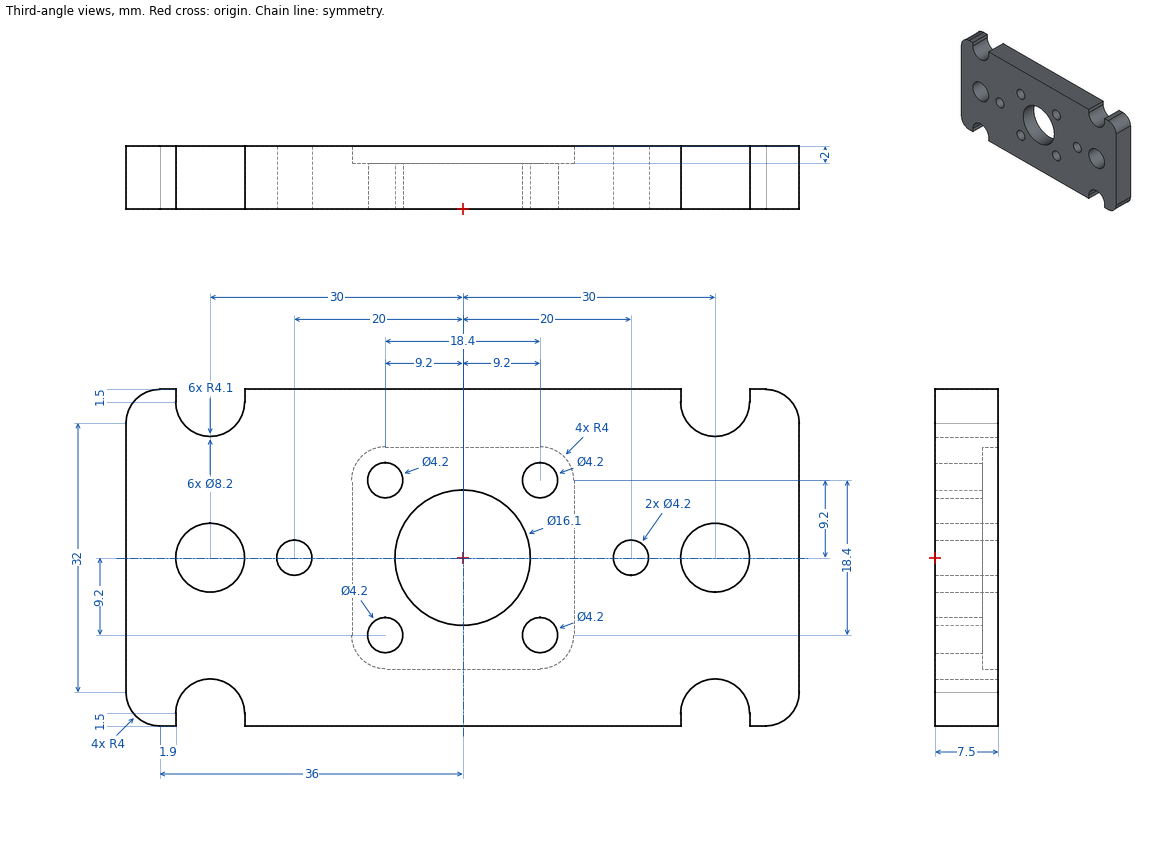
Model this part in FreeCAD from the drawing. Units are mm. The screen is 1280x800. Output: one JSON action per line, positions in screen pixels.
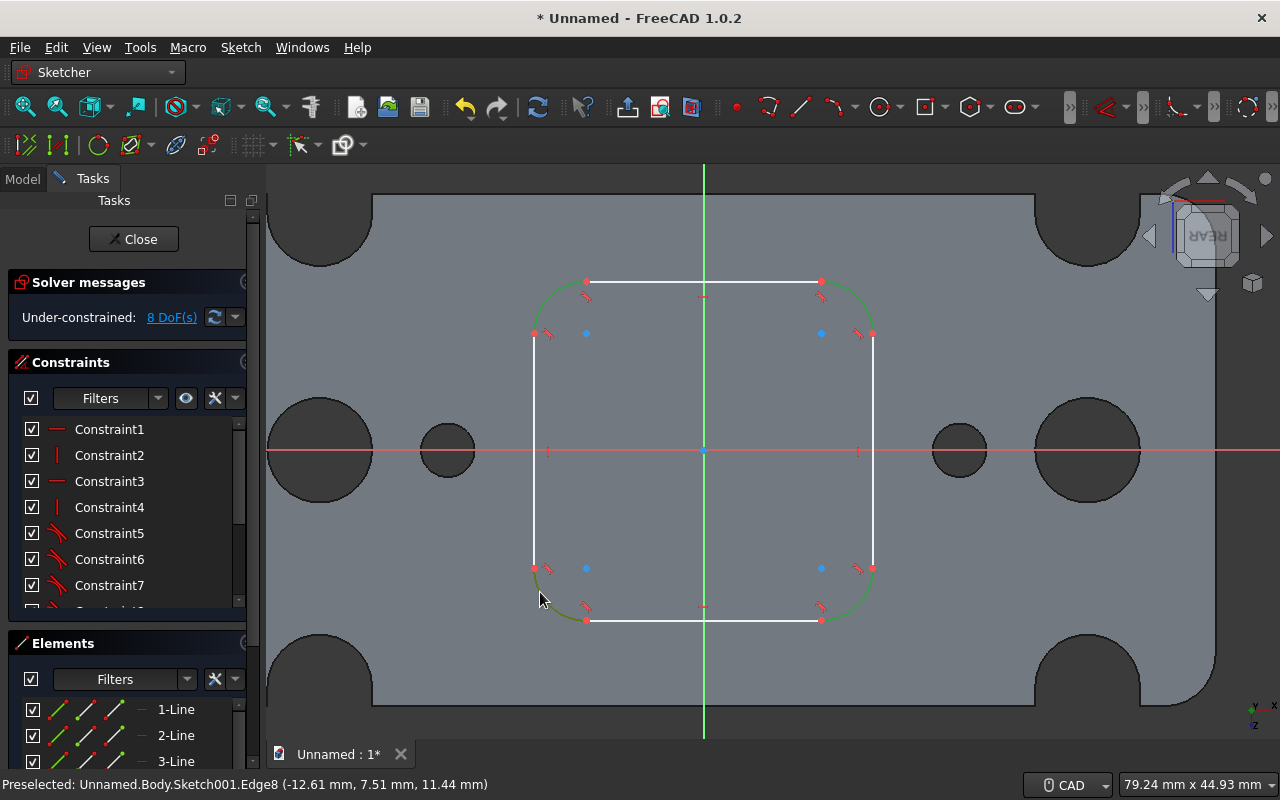
{"action": "key", "text": "e"}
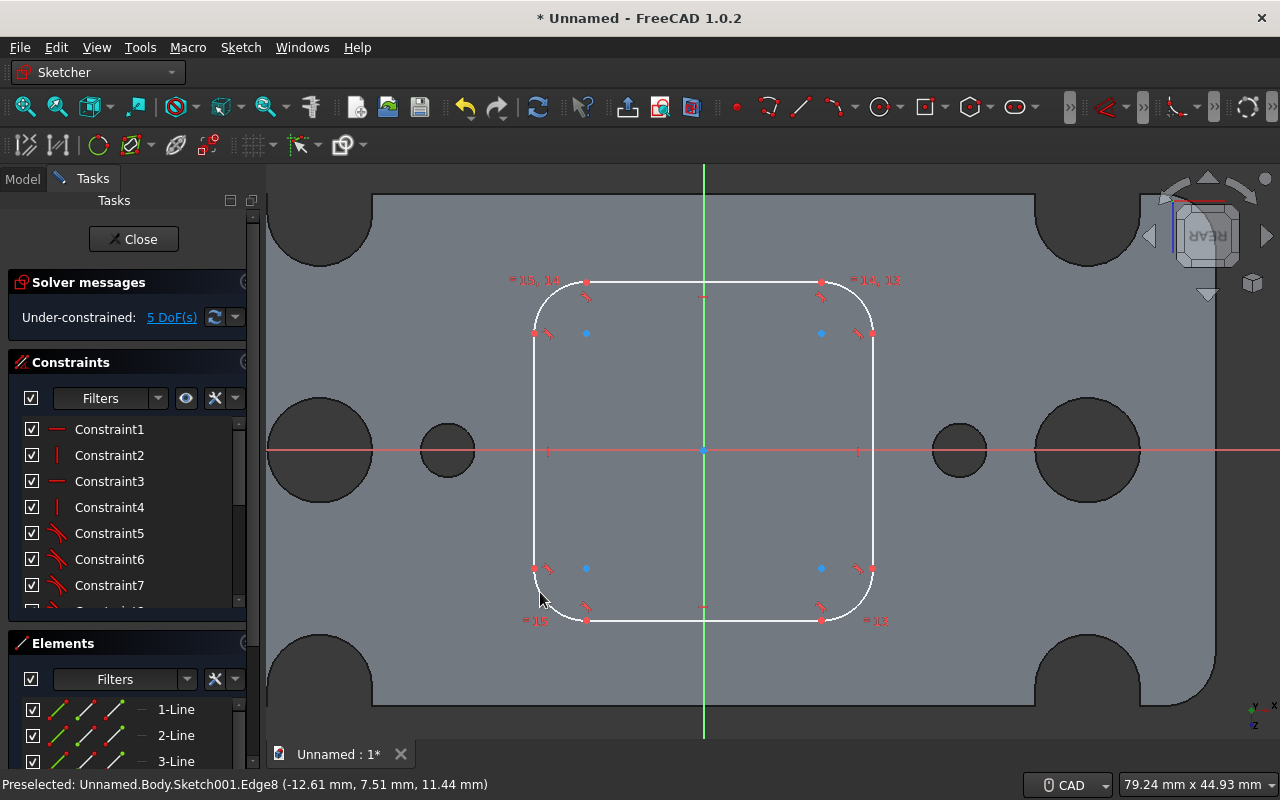
{"action": "left_click", "coordinate": [1106, 108]}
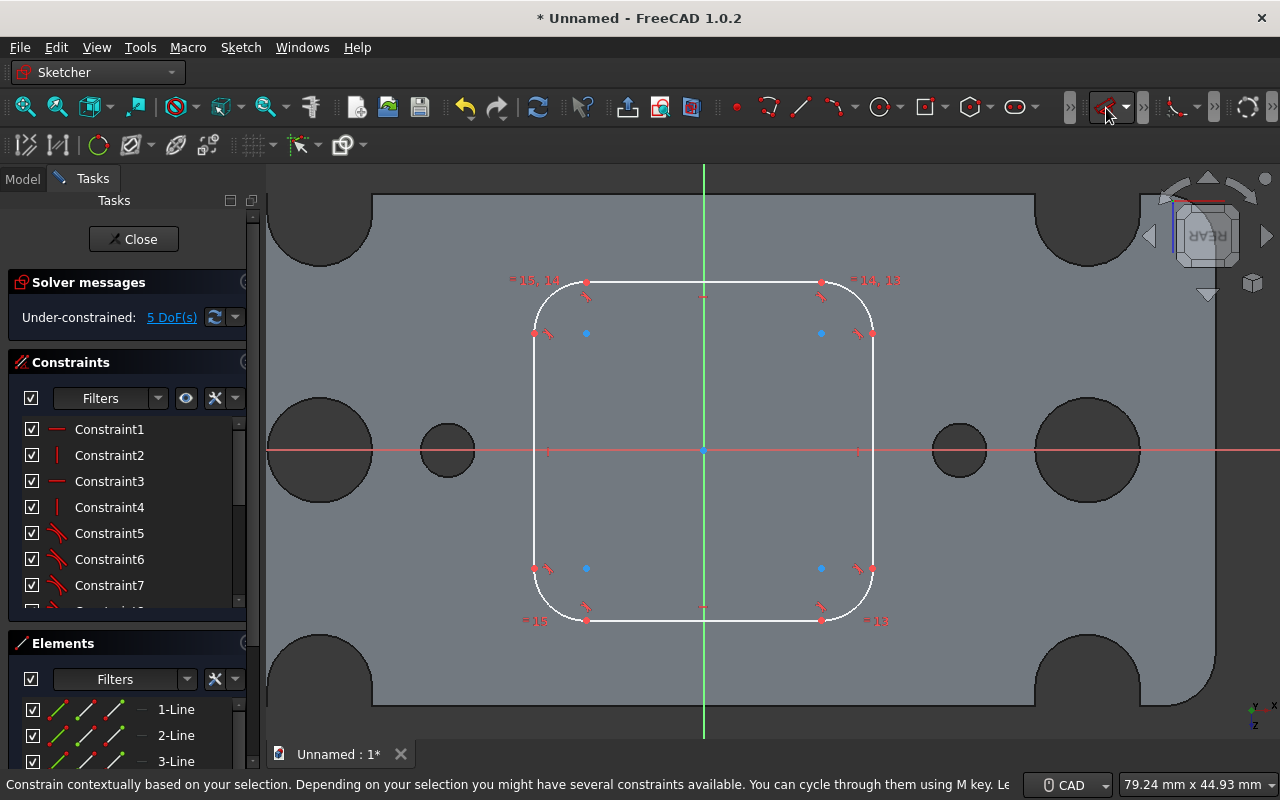
{"action": "left_click", "coordinate": [845, 615]}
{"action": "left_click", "coordinate": [860, 643]}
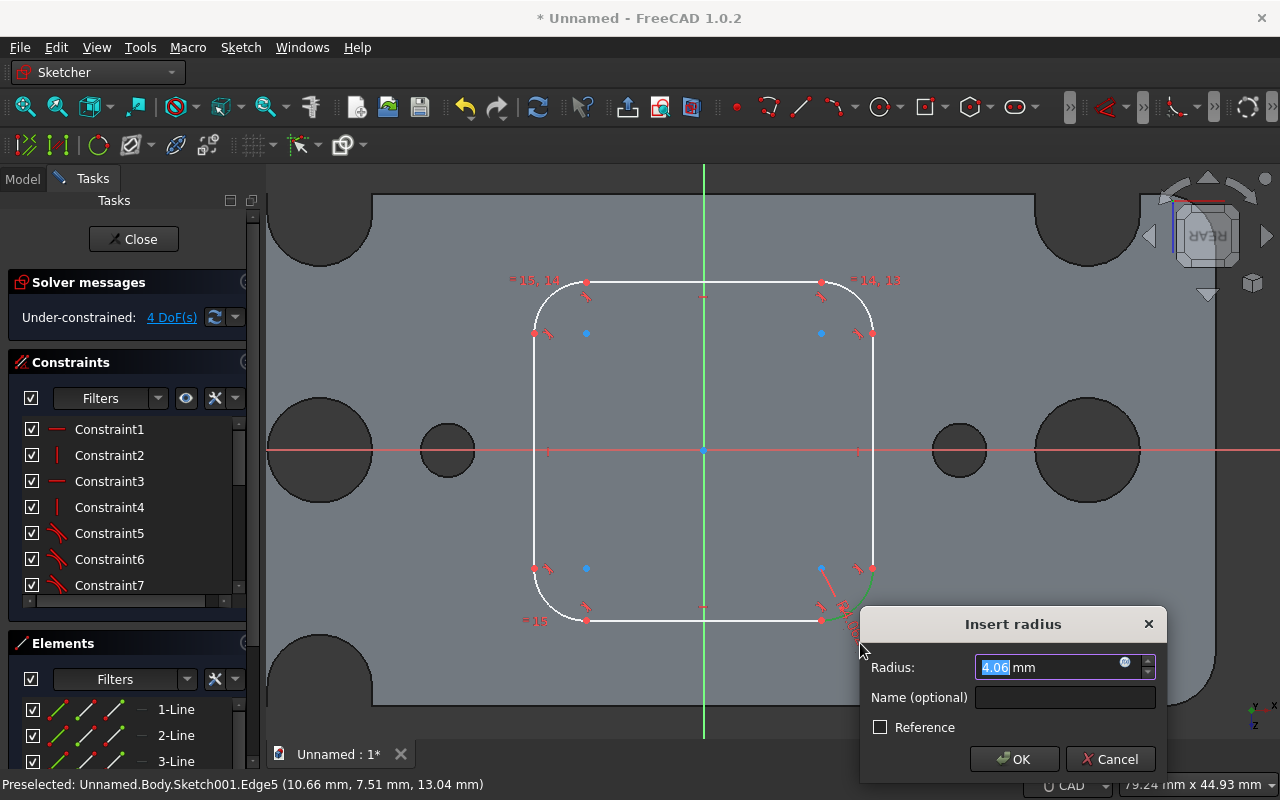
{"action": "type", "text": "4"}
{"action": "key", "text": "Return"}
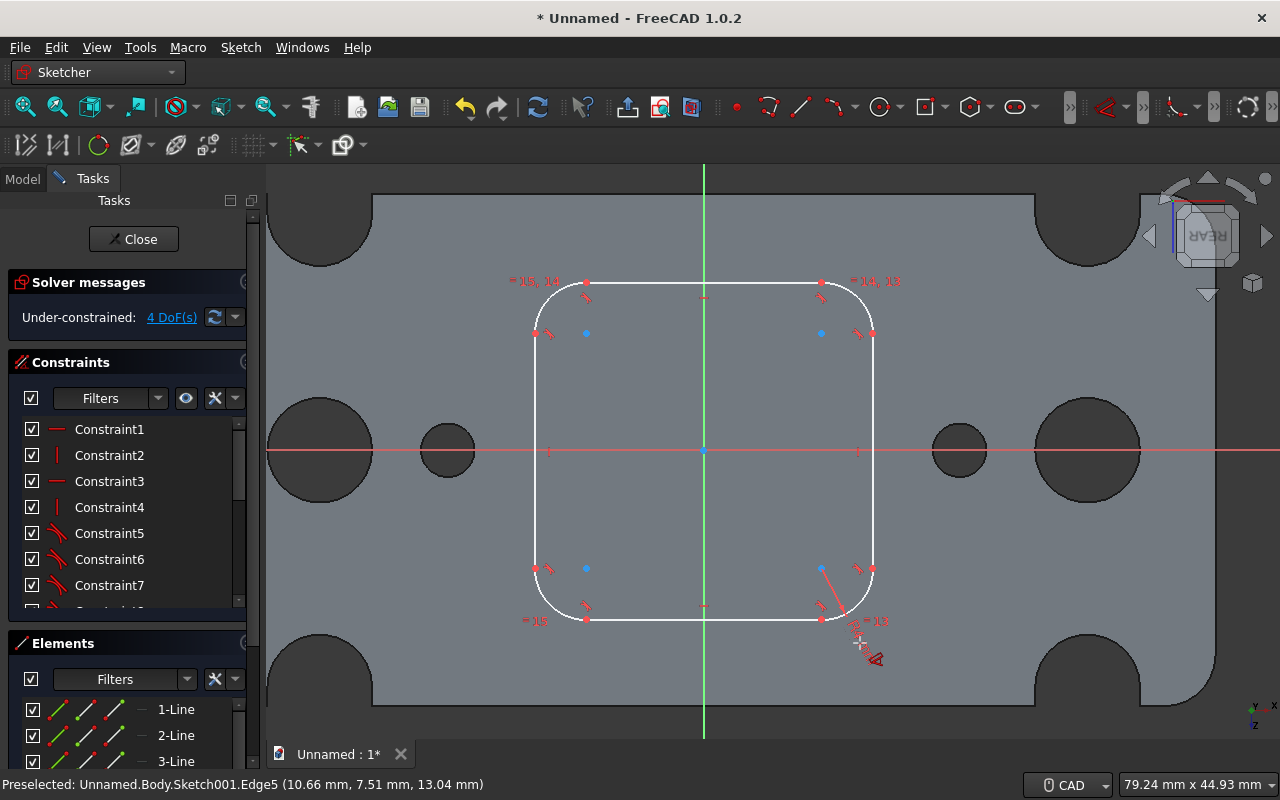
{"action": "left_click", "coordinate": [657, 620]}
{"action": "left_click", "coordinate": [650, 654]}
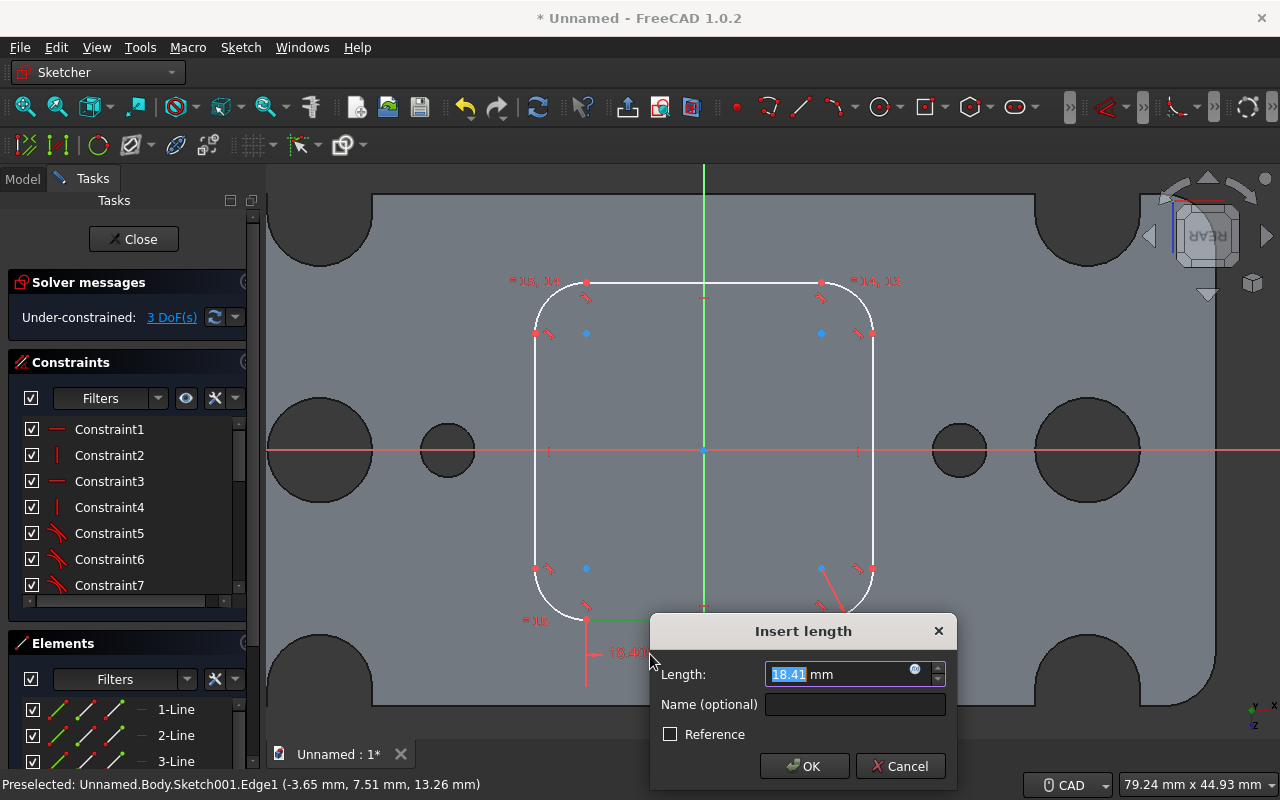
{"action": "type", "text": "18.4"}
{"action": "key", "text": "Return"}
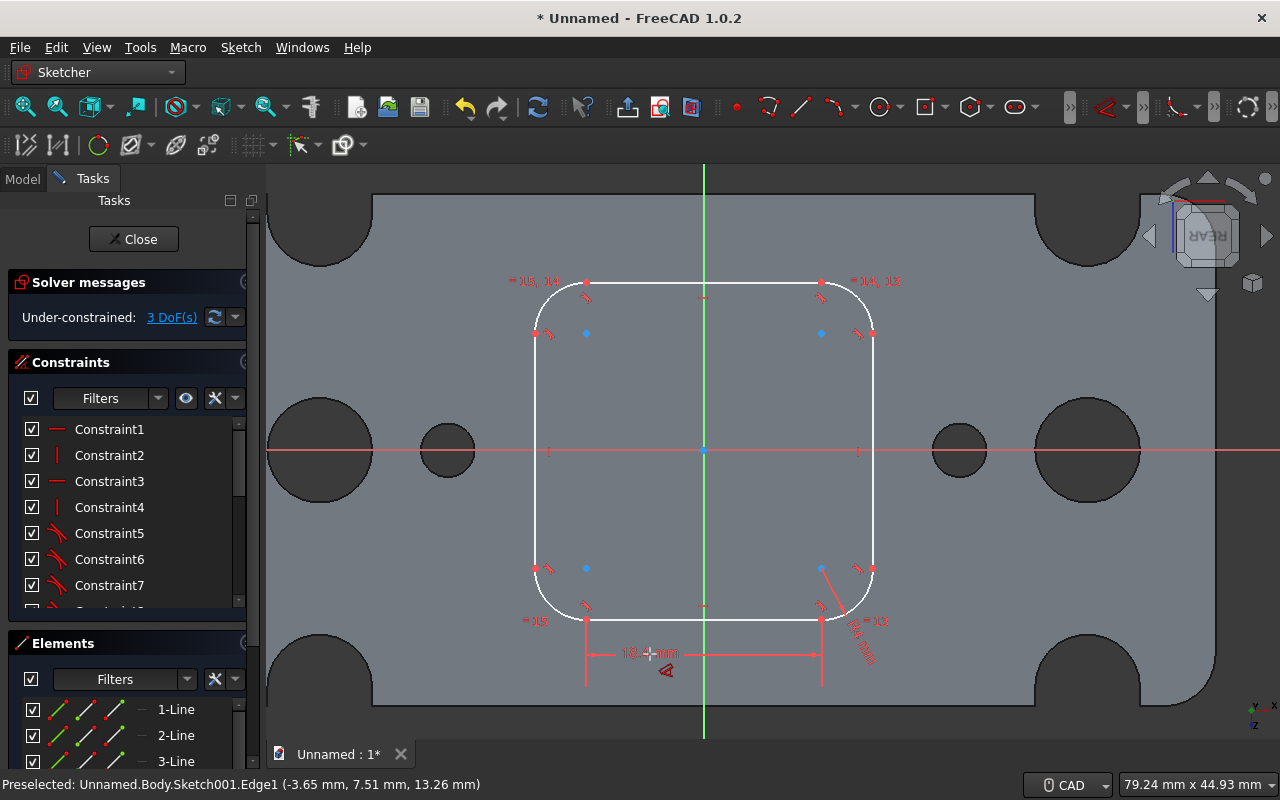
{"action": "left_click", "coordinate": [873, 498]}
{"action": "left_click", "coordinate": [907, 397]}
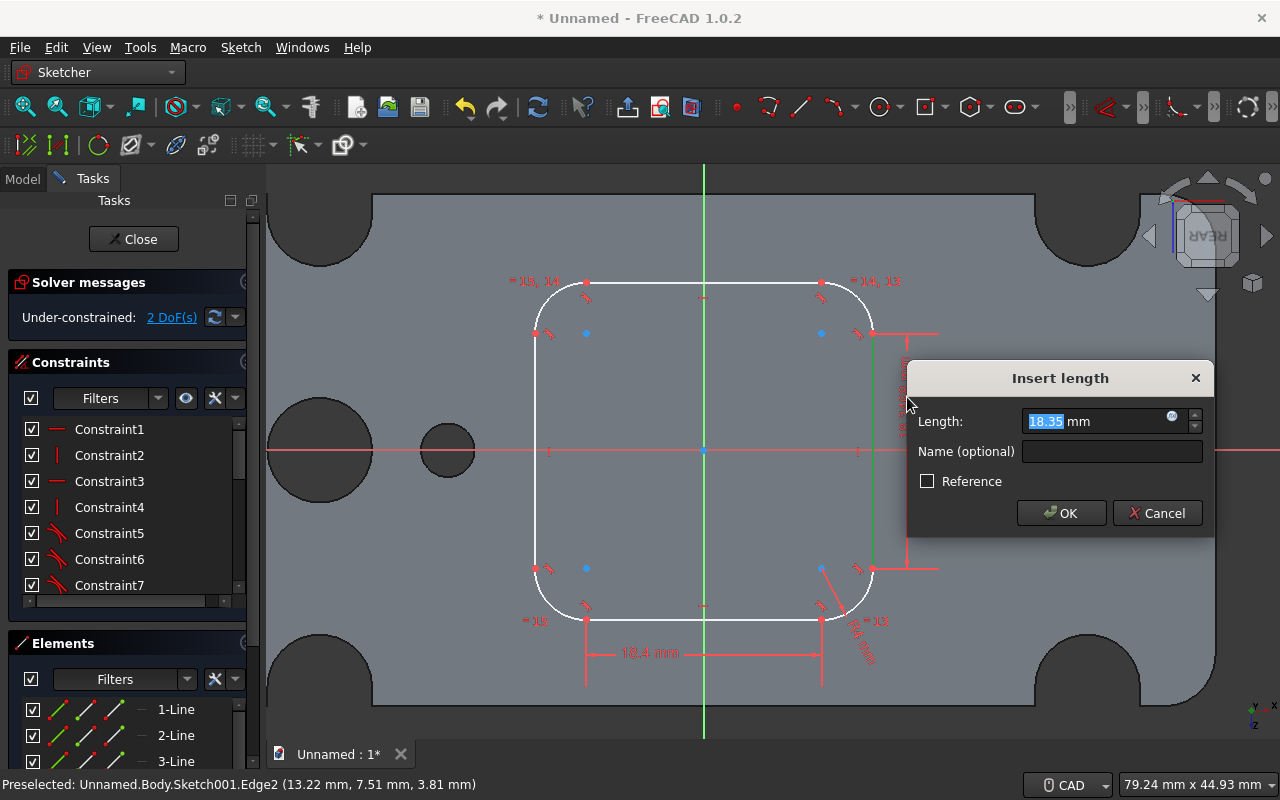
{"action": "type", "text": "18.4"}
{"action": "key", "text": "Return"}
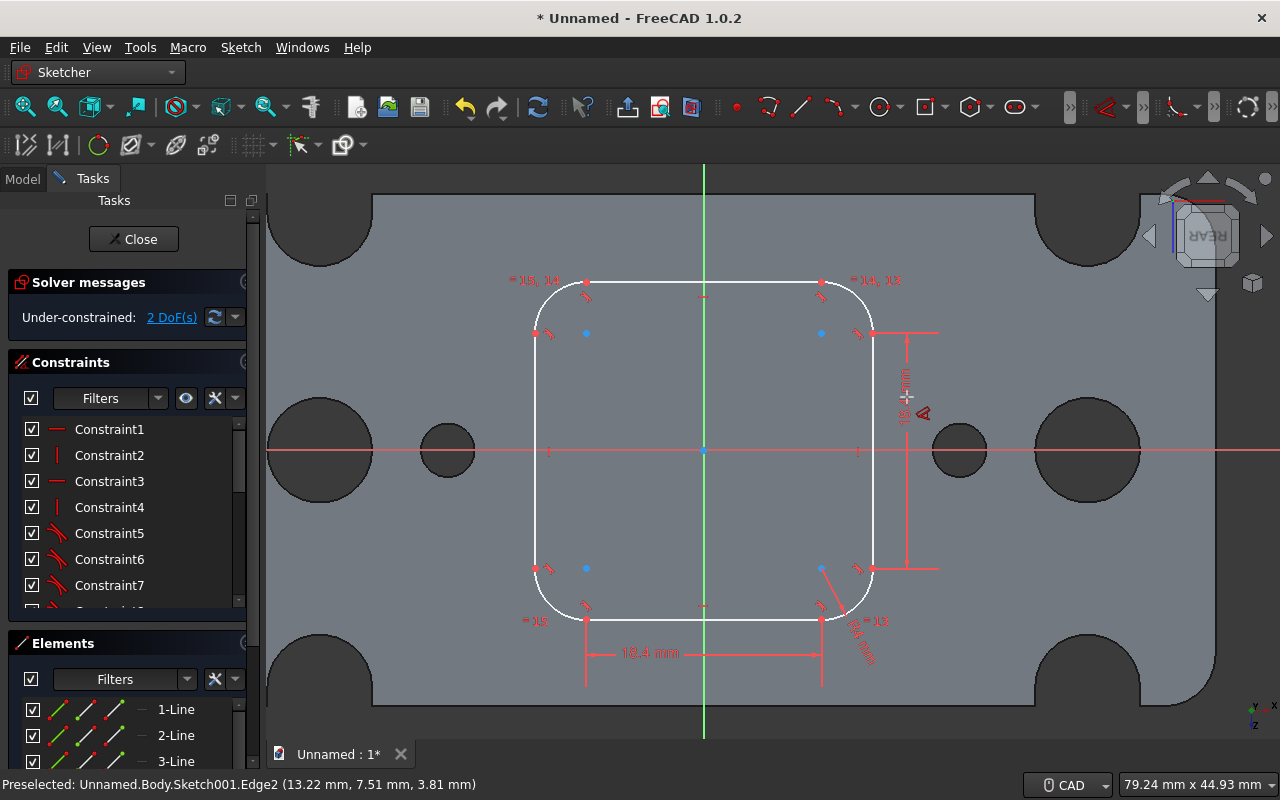
{"action": "left_click", "coordinate": [586, 620]}
{"action": "left_click", "coordinate": [645, 416]}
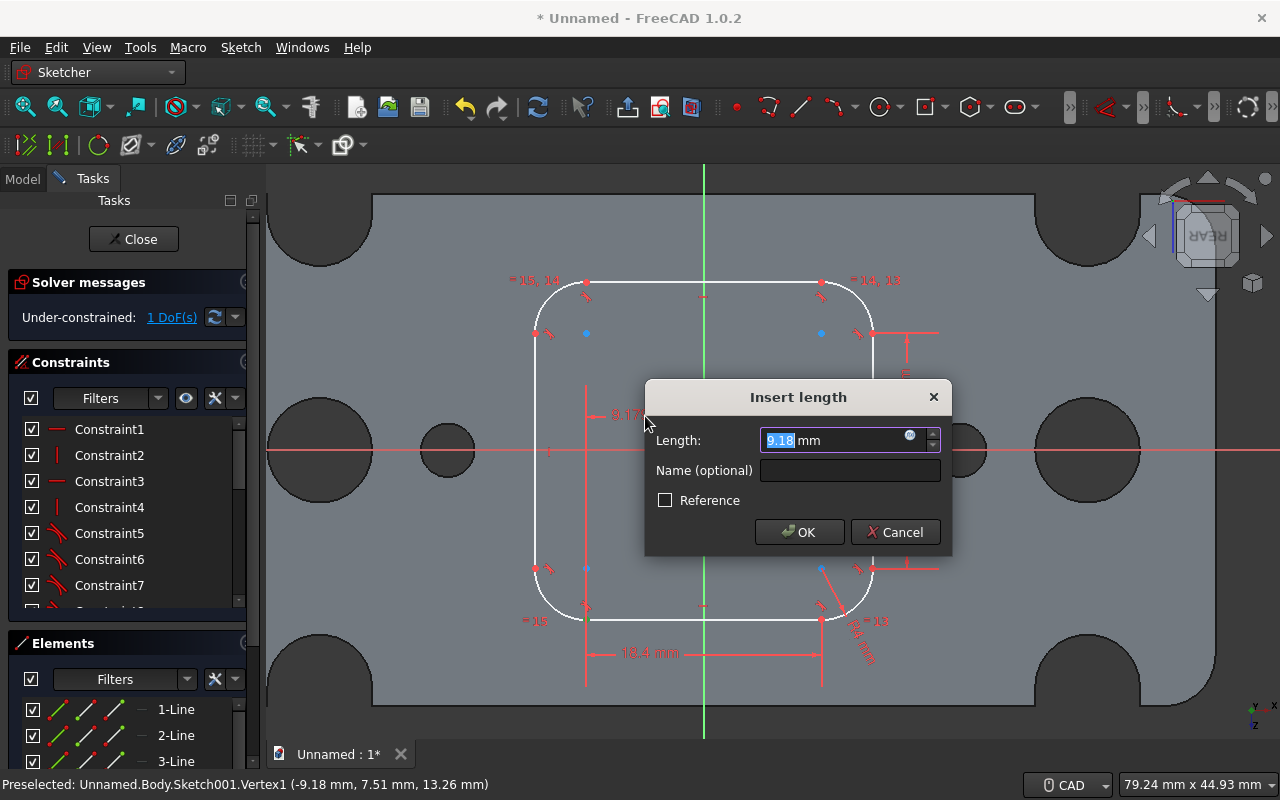
{"action": "type", "text": "9.2"}
{"action": "key", "text": "Return"}